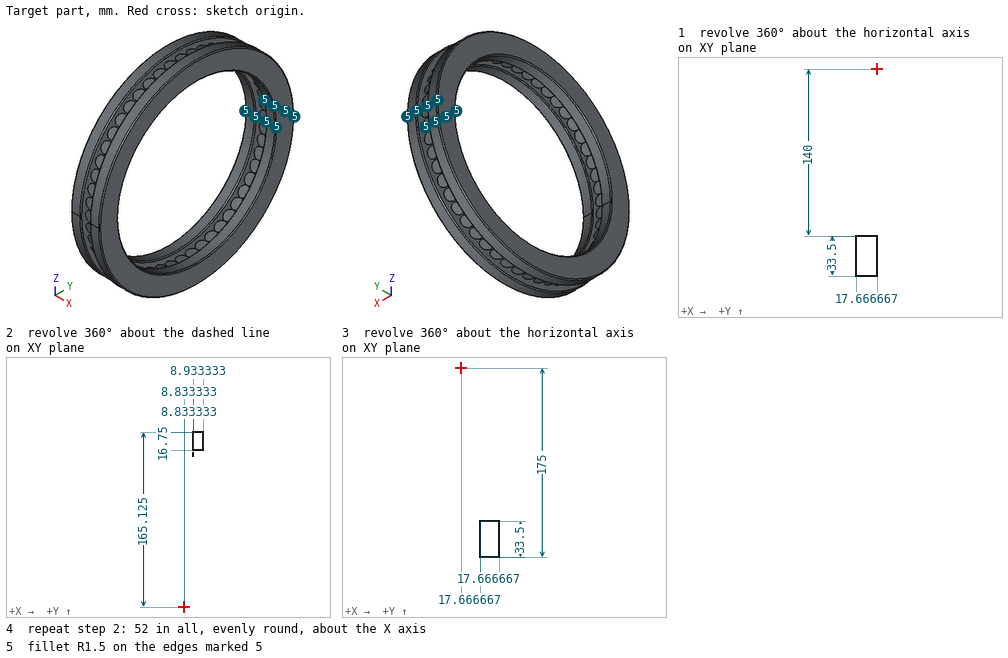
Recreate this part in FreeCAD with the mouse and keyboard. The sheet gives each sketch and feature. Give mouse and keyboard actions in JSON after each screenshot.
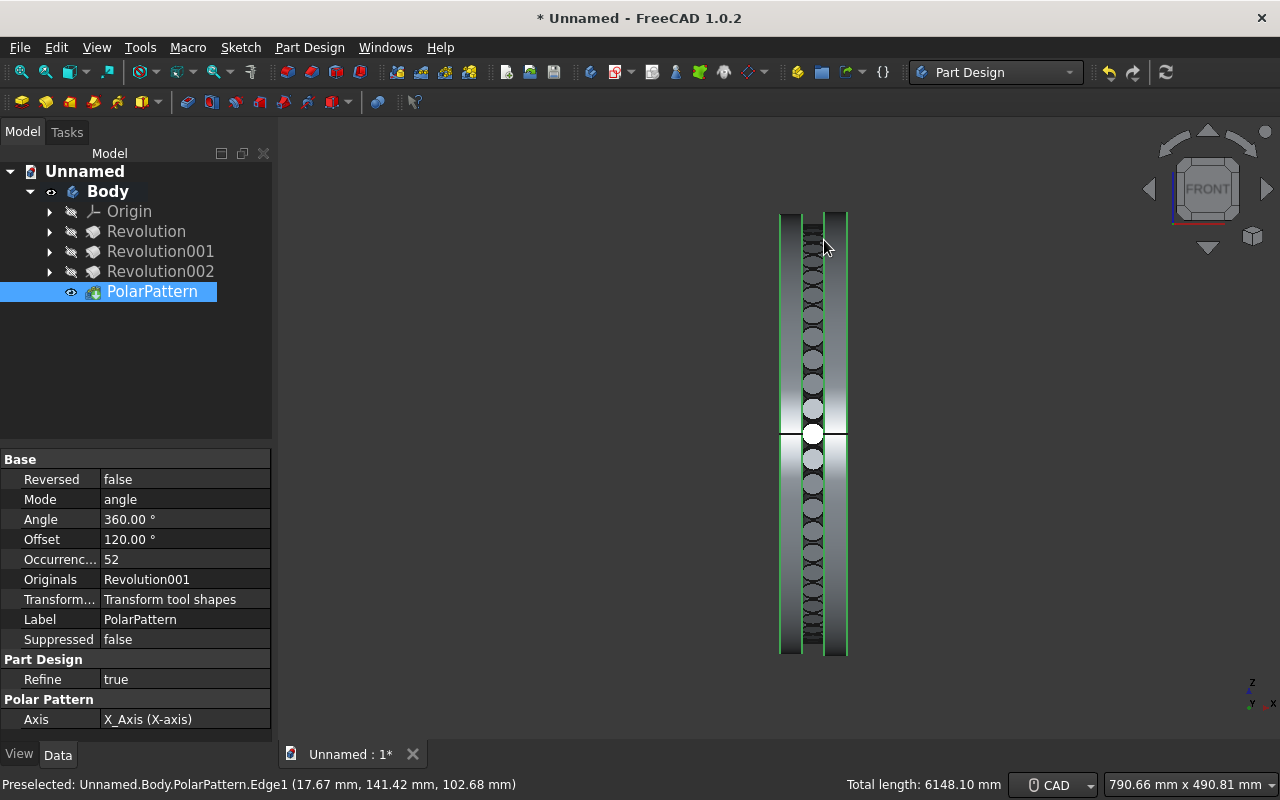
{"action": "key", "text": "3"}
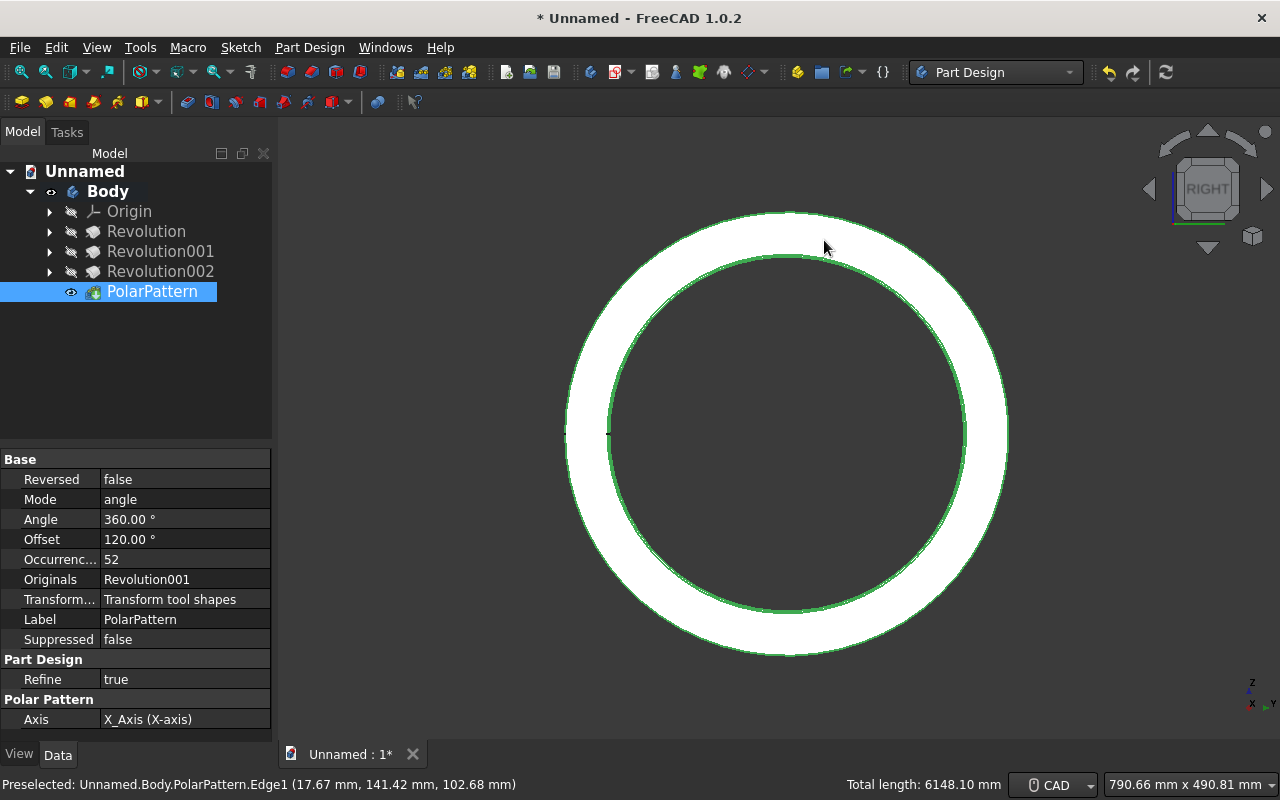
{"action": "key", "text": "5"}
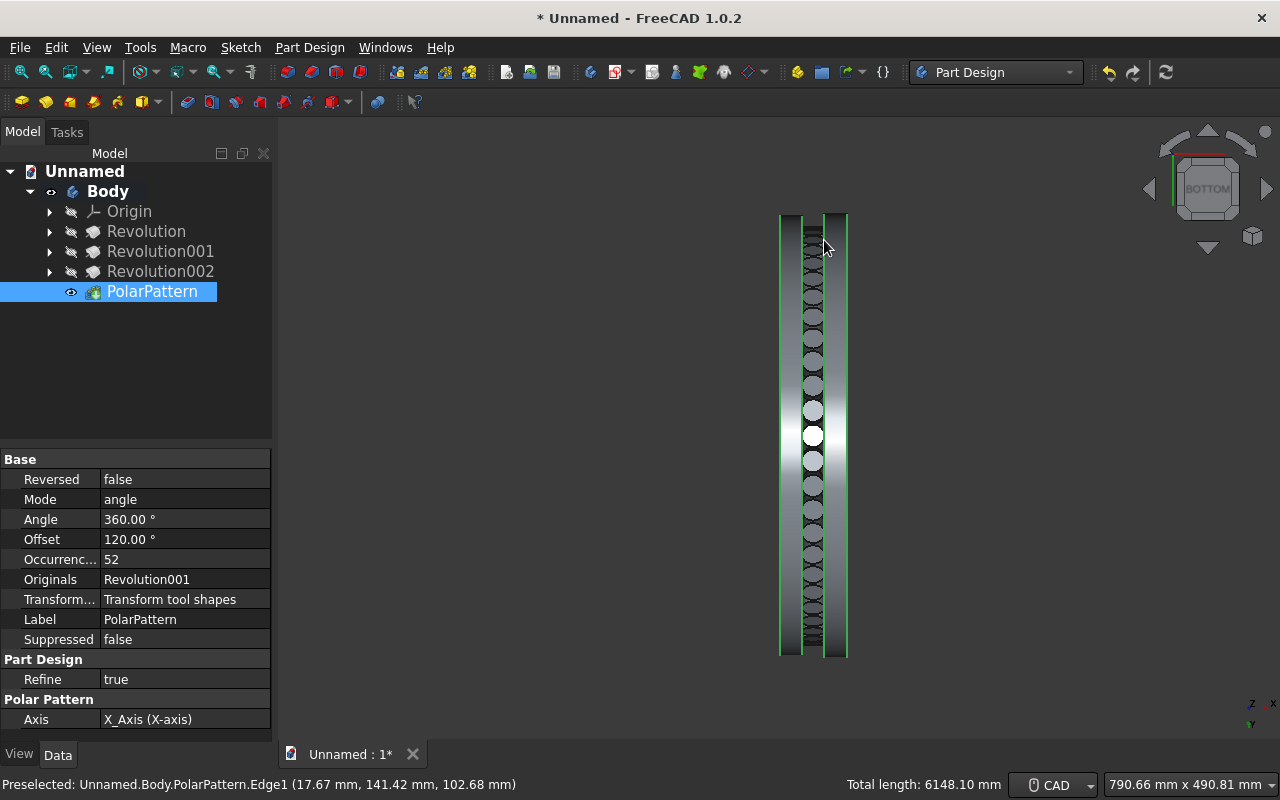
{"action": "key", "text": "4"}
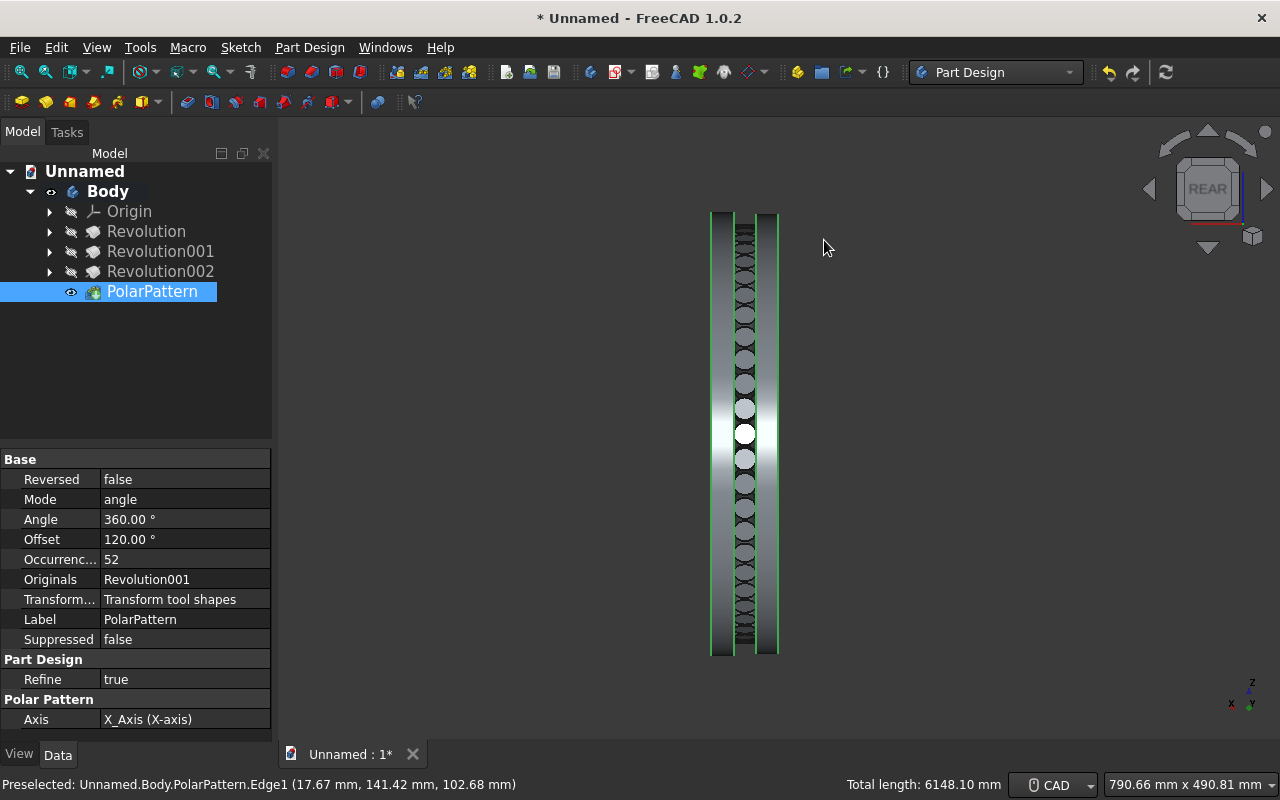
{"action": "key", "text": "6"}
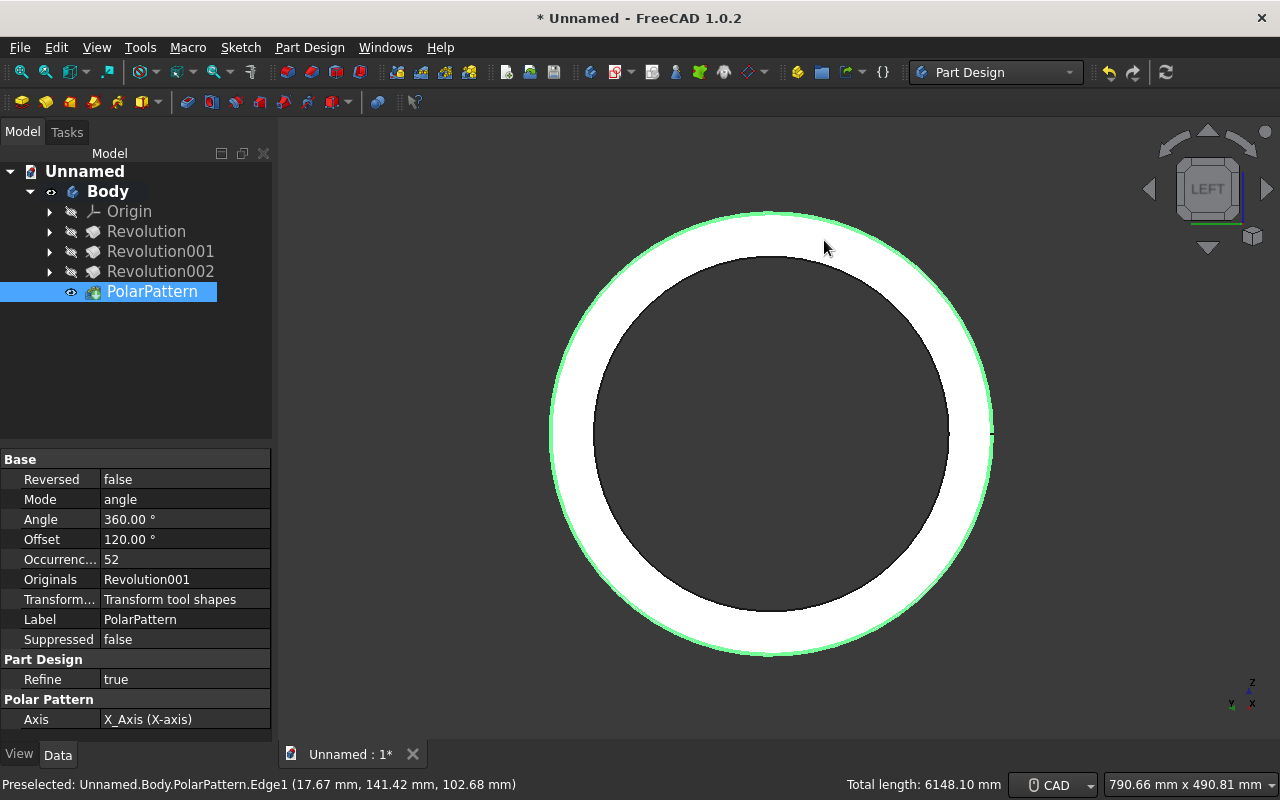
{"action": "left_click", "coordinate": [594, 433], "text": "ctrl"}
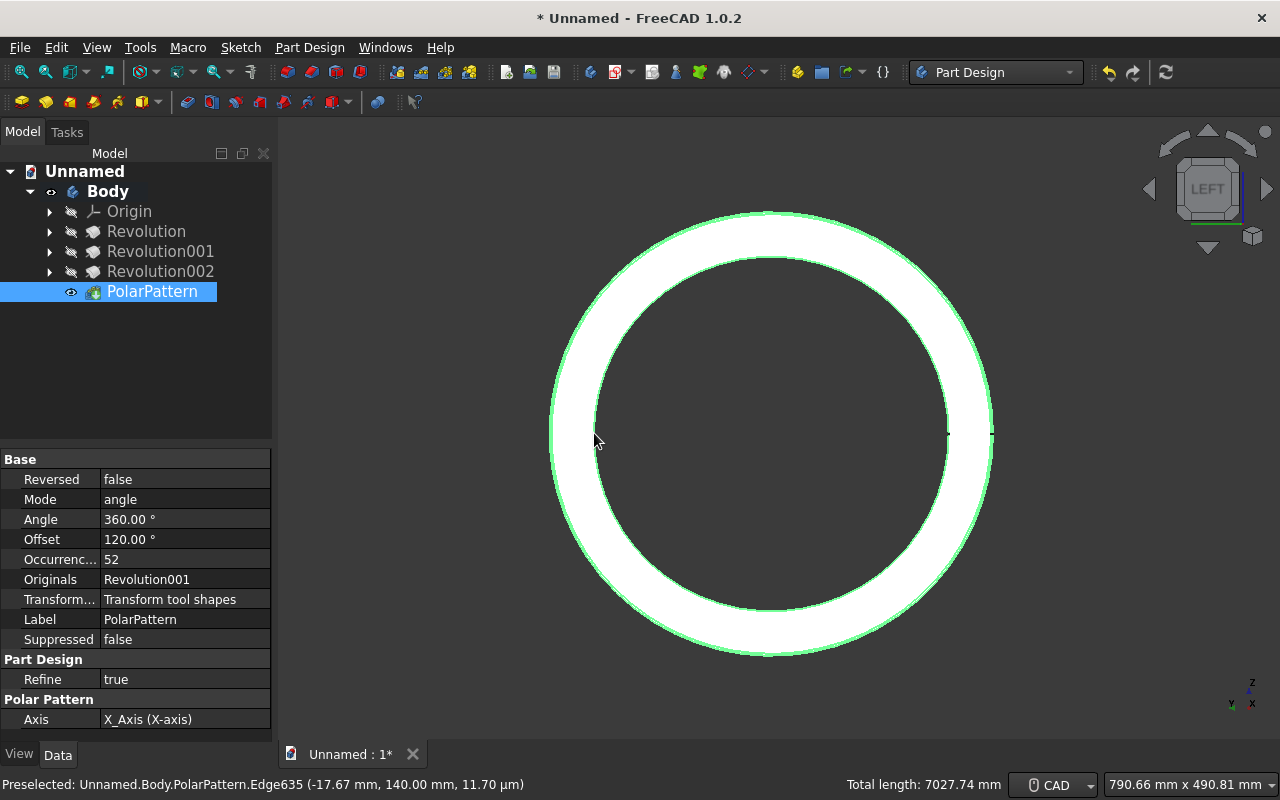
{"action": "key", "text": "v 3"}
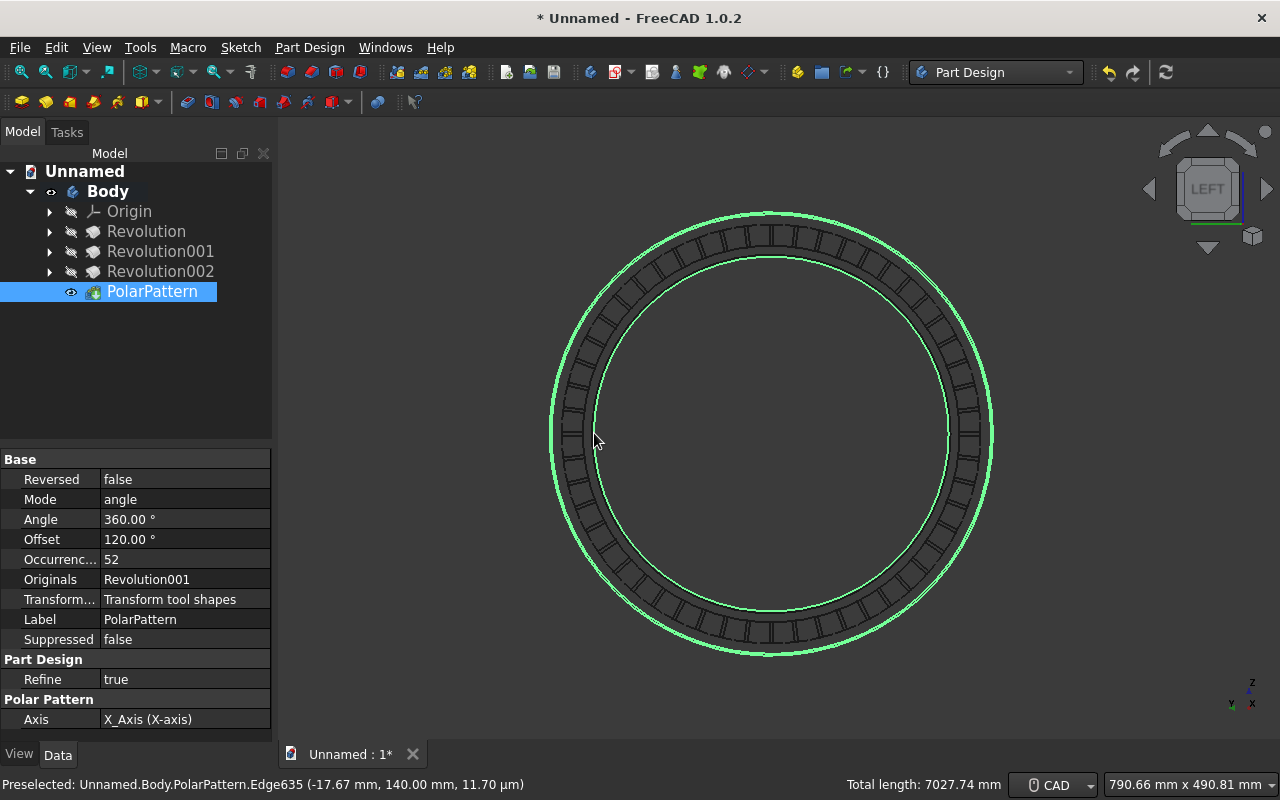
{"action": "key", "text": "0"}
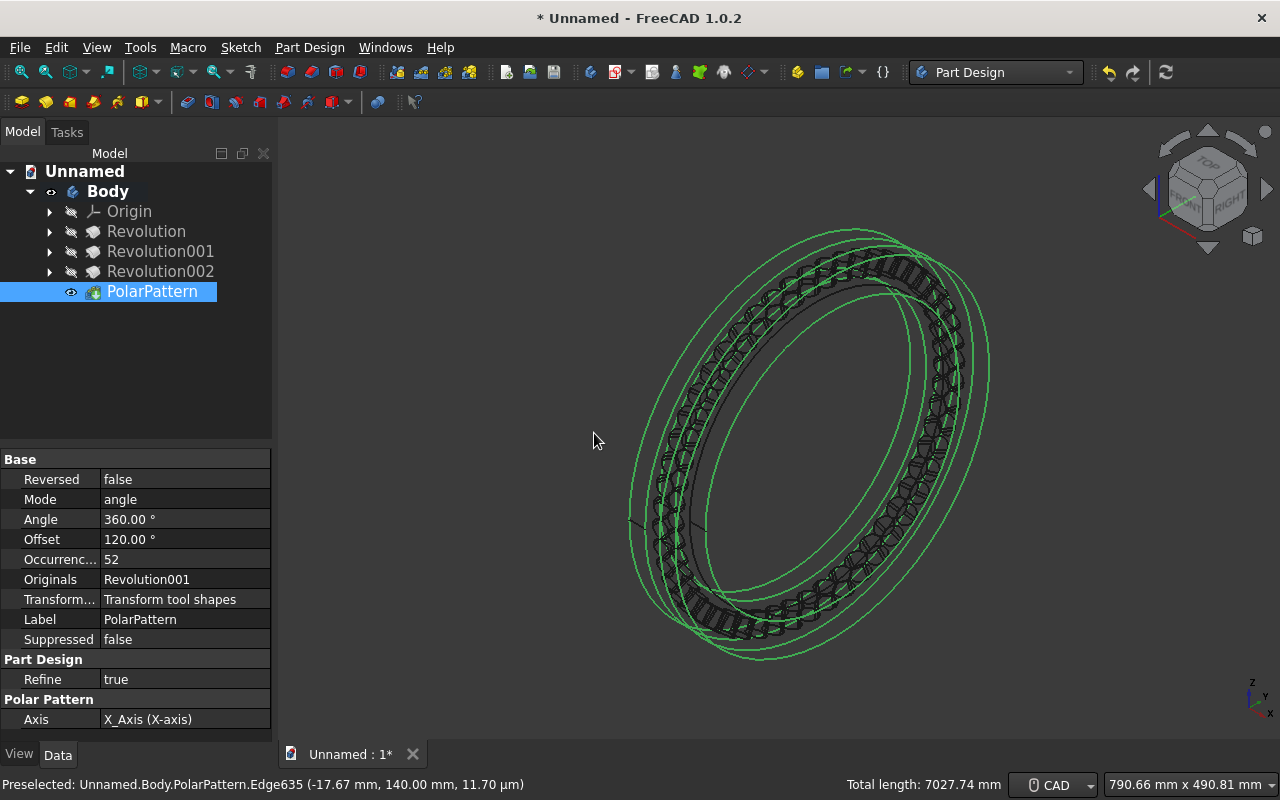
{"action": "left_click", "coordinate": [943, 374], "text": "ctrl"}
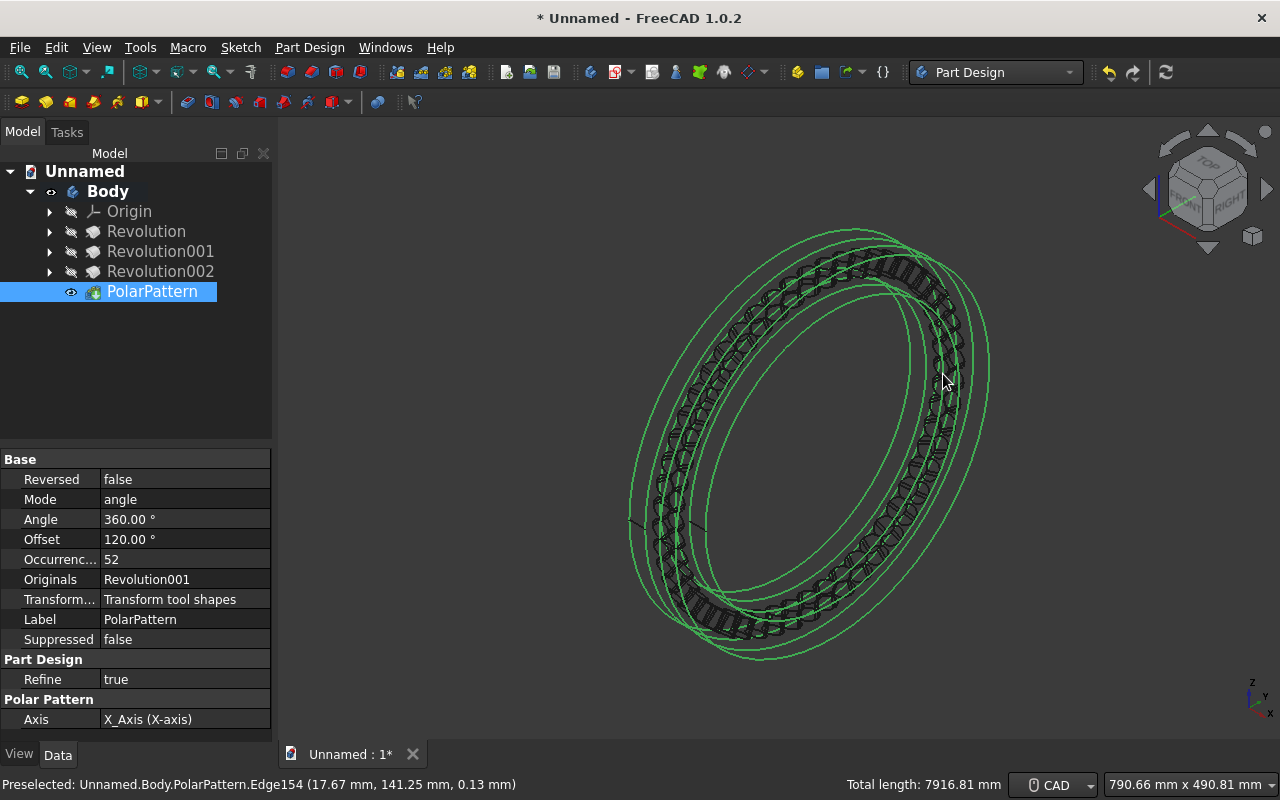
{"action": "key", "text": "v 1"}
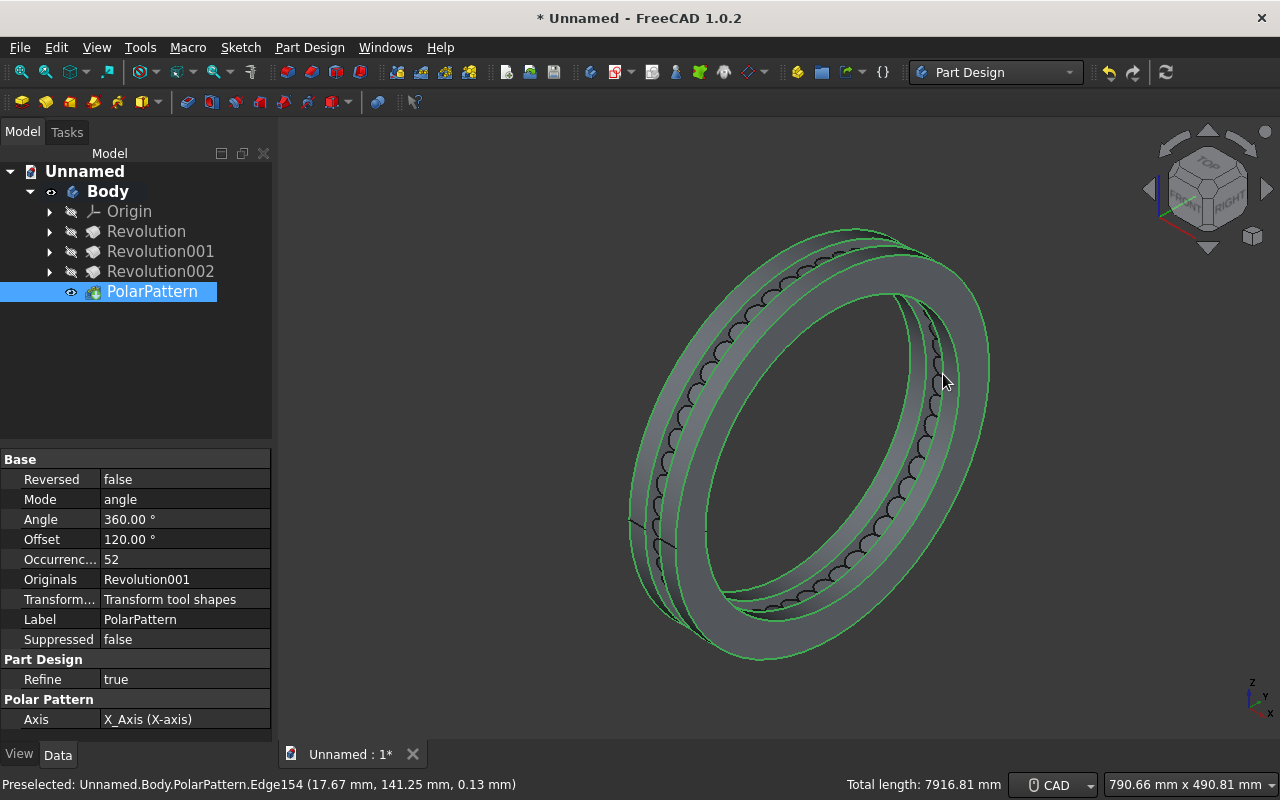
{"action": "left_click", "coordinate": [288, 72]}